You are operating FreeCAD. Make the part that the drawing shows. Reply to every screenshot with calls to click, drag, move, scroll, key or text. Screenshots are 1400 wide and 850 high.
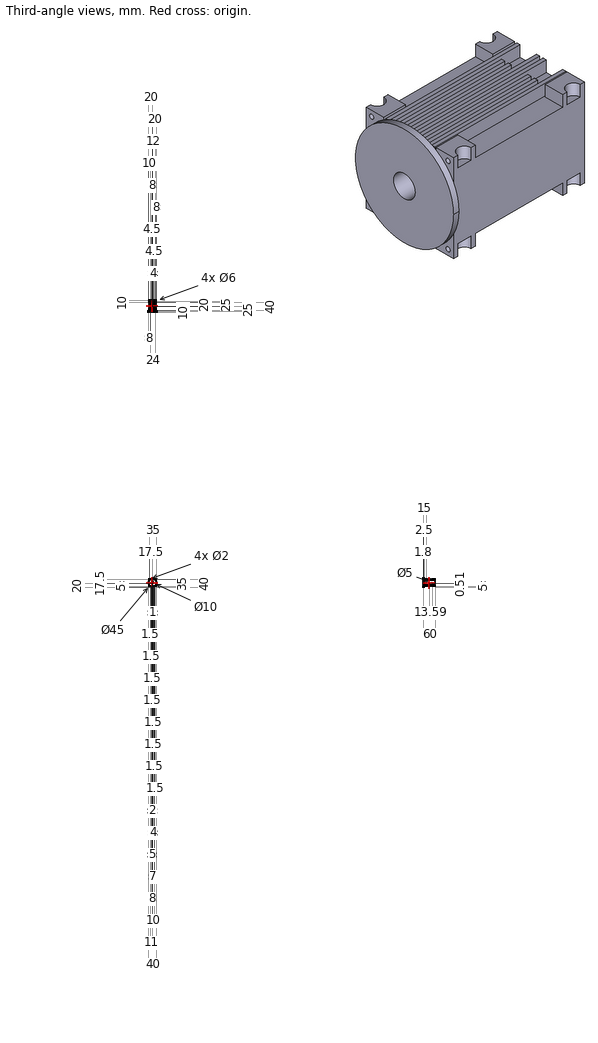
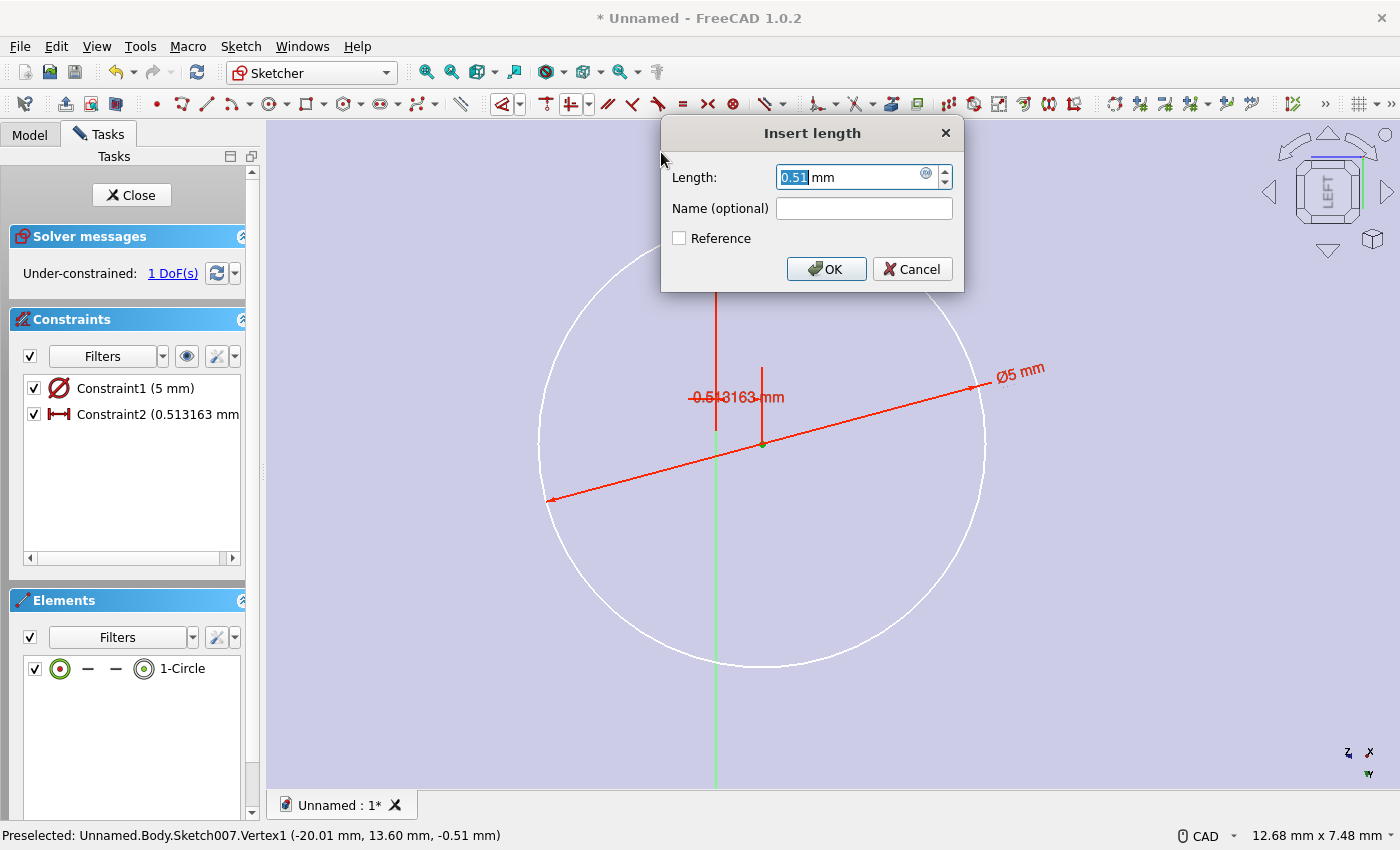
text(0.51)
key(Return)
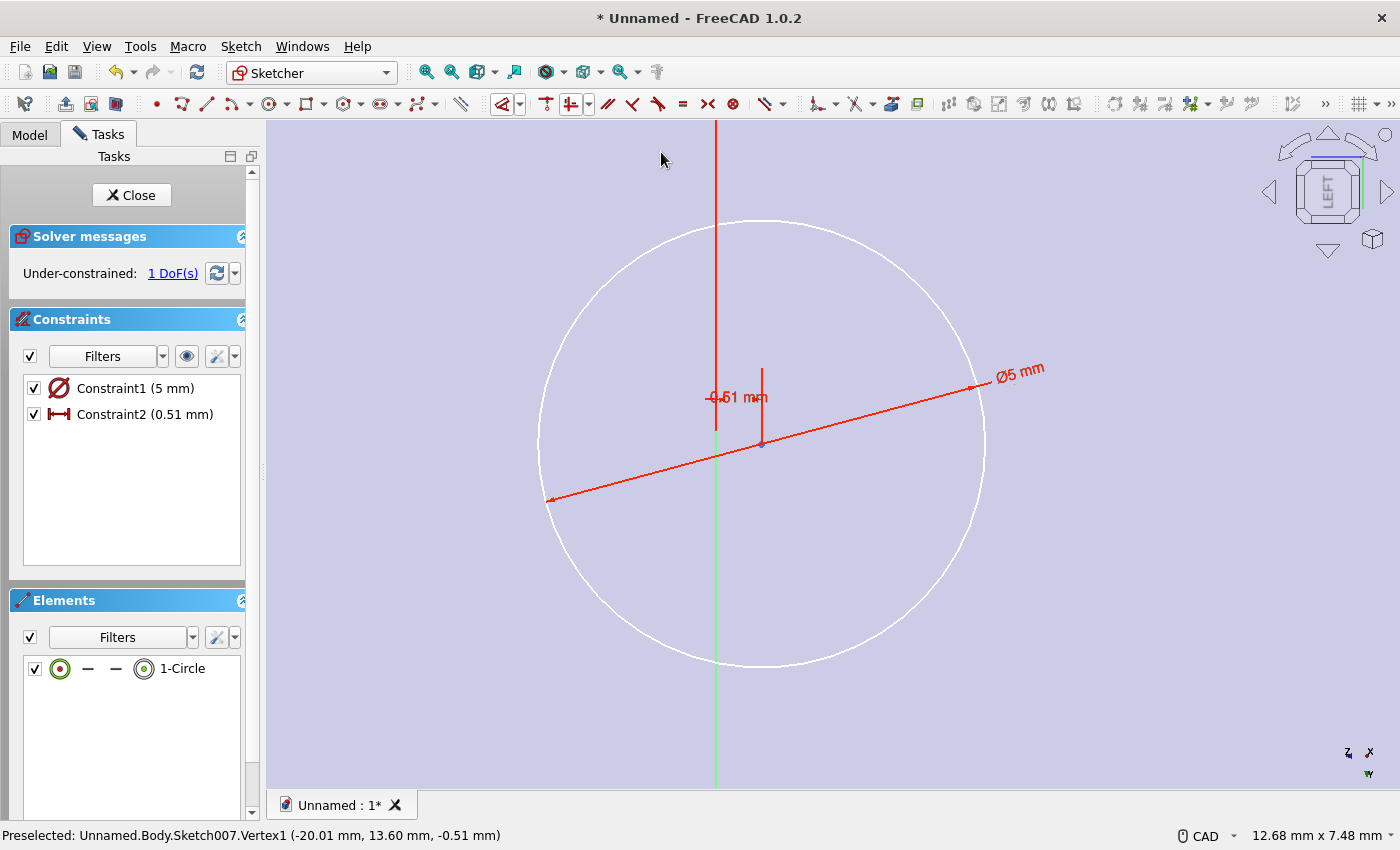
click(762, 444)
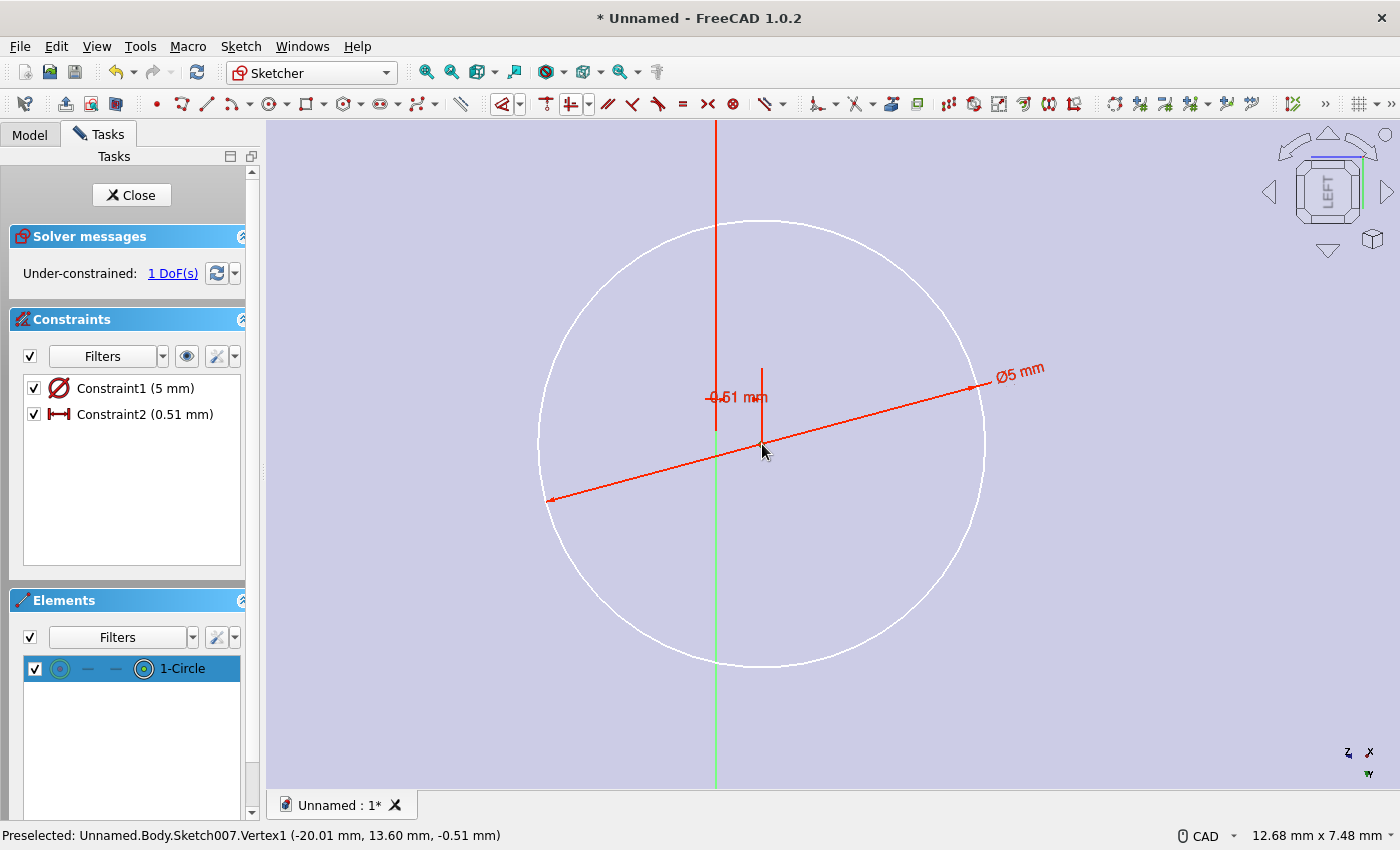
click(520, 104)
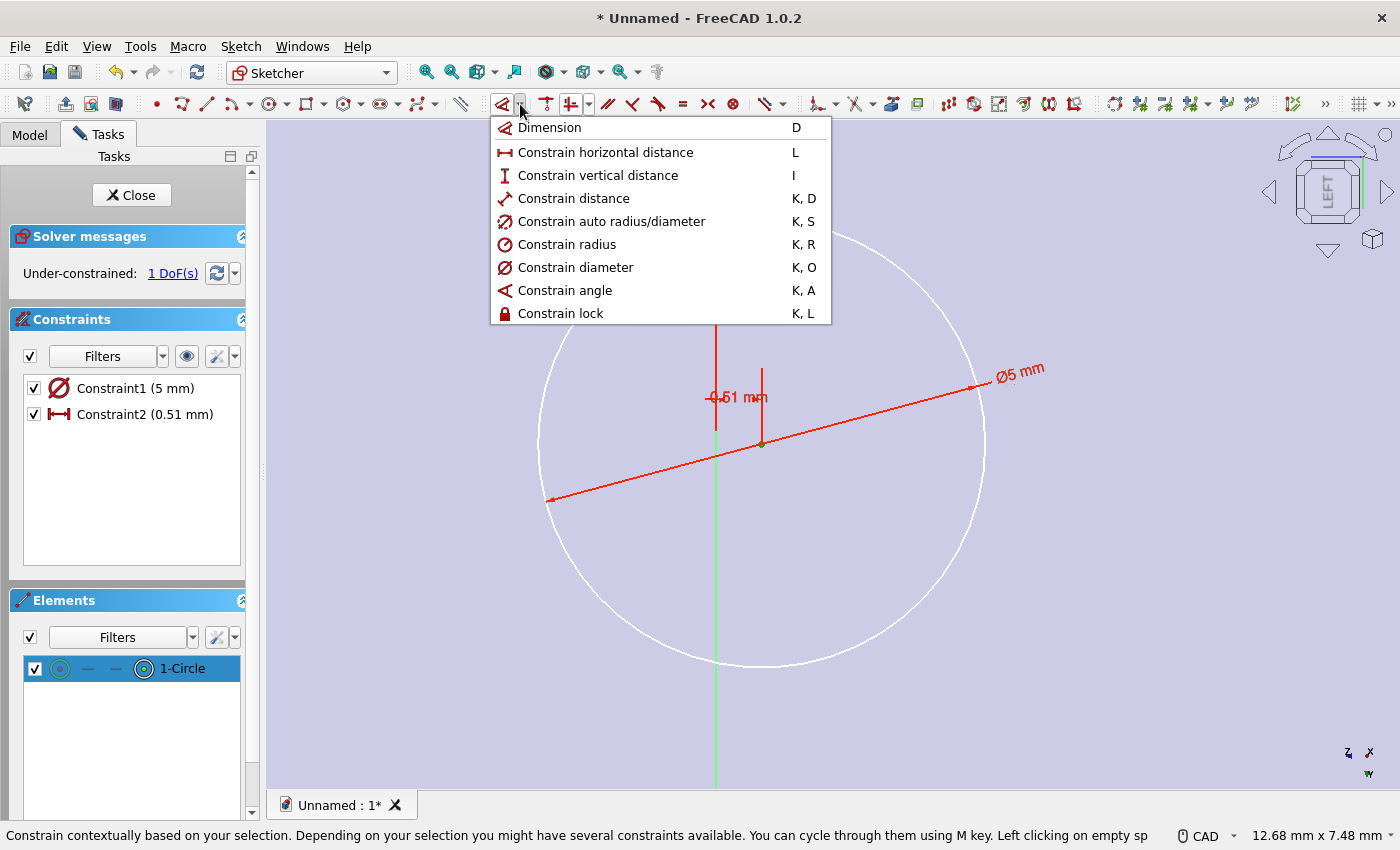
click(661, 176)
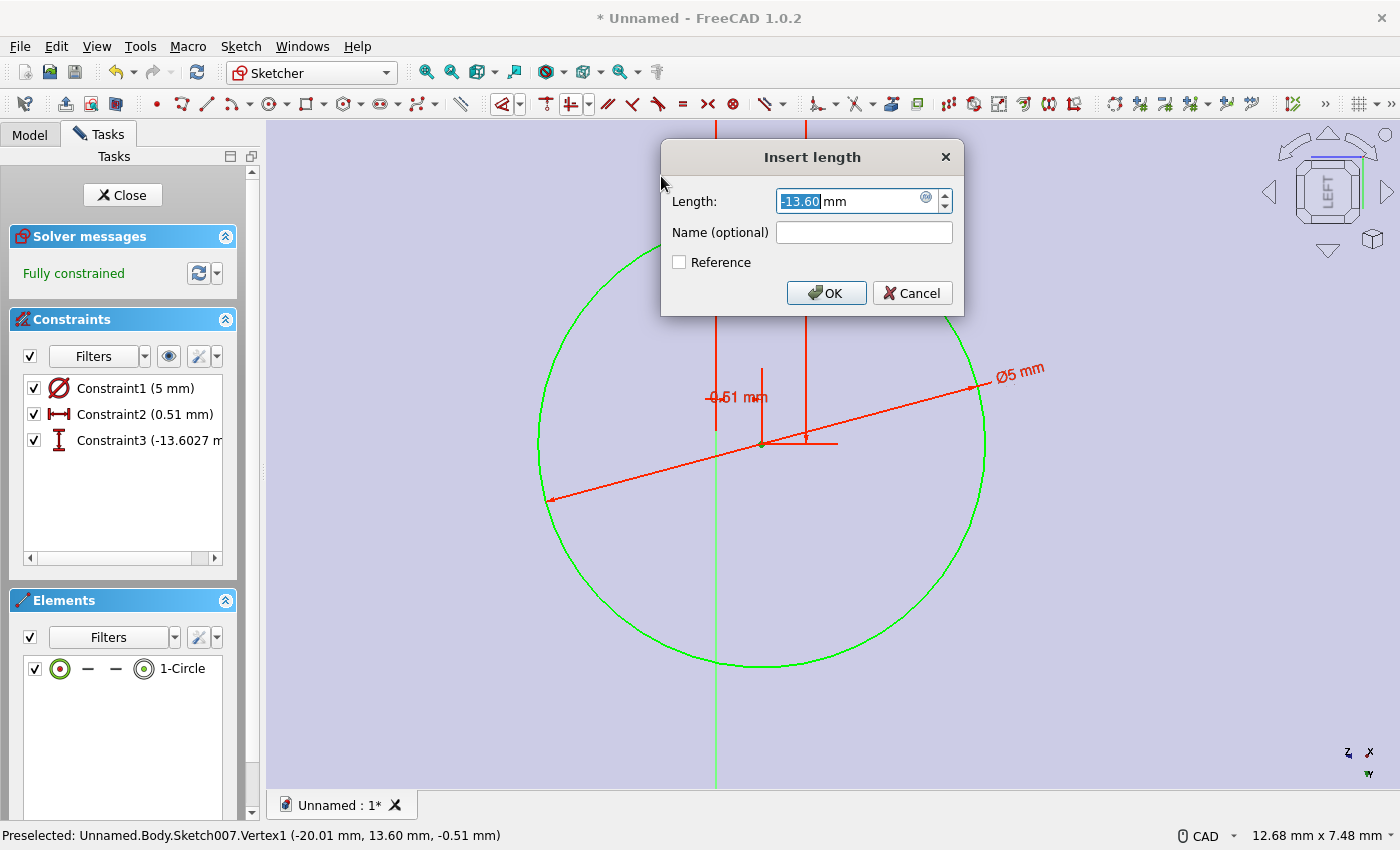
text(-13.59)
key(Return)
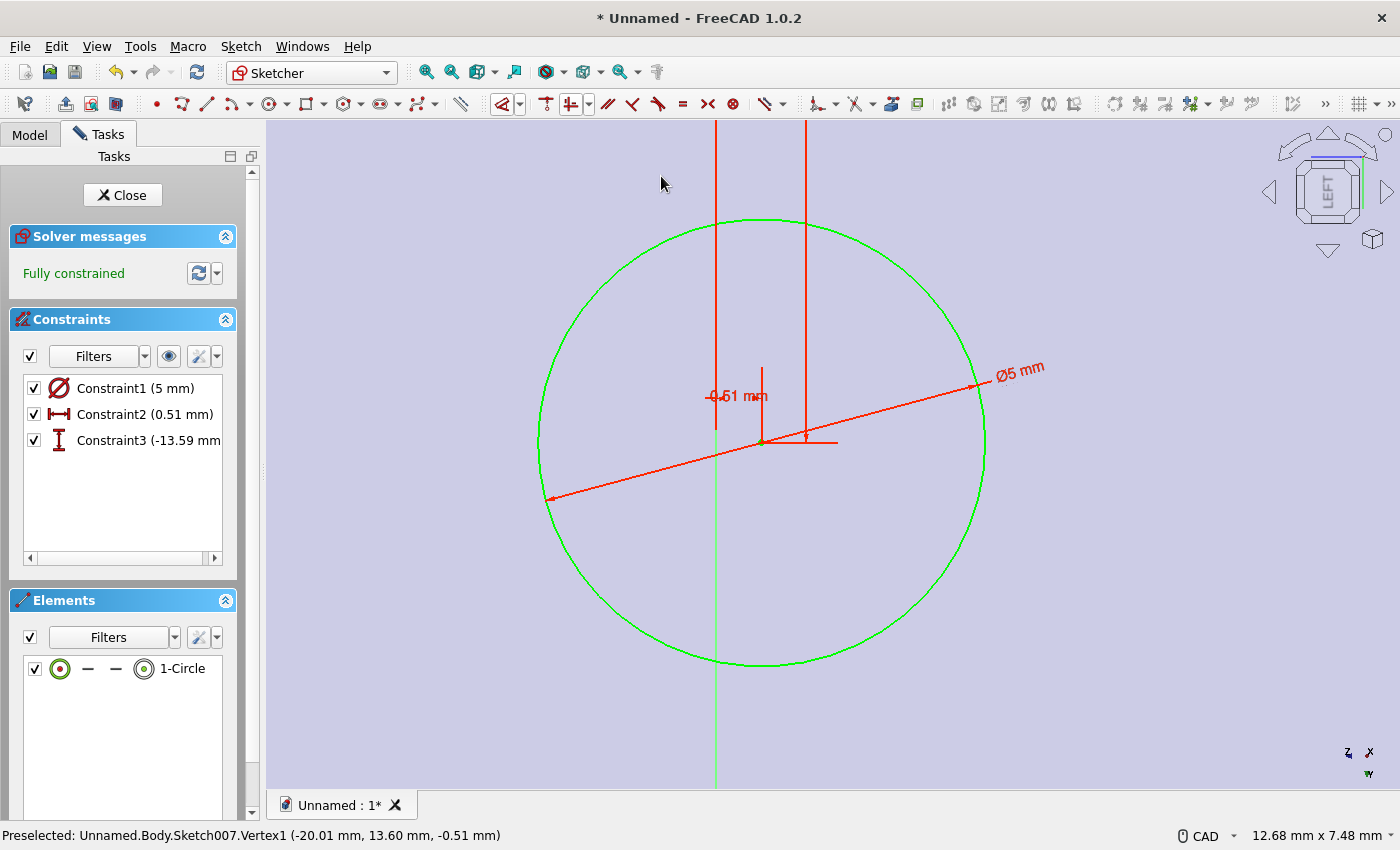
click(123, 195)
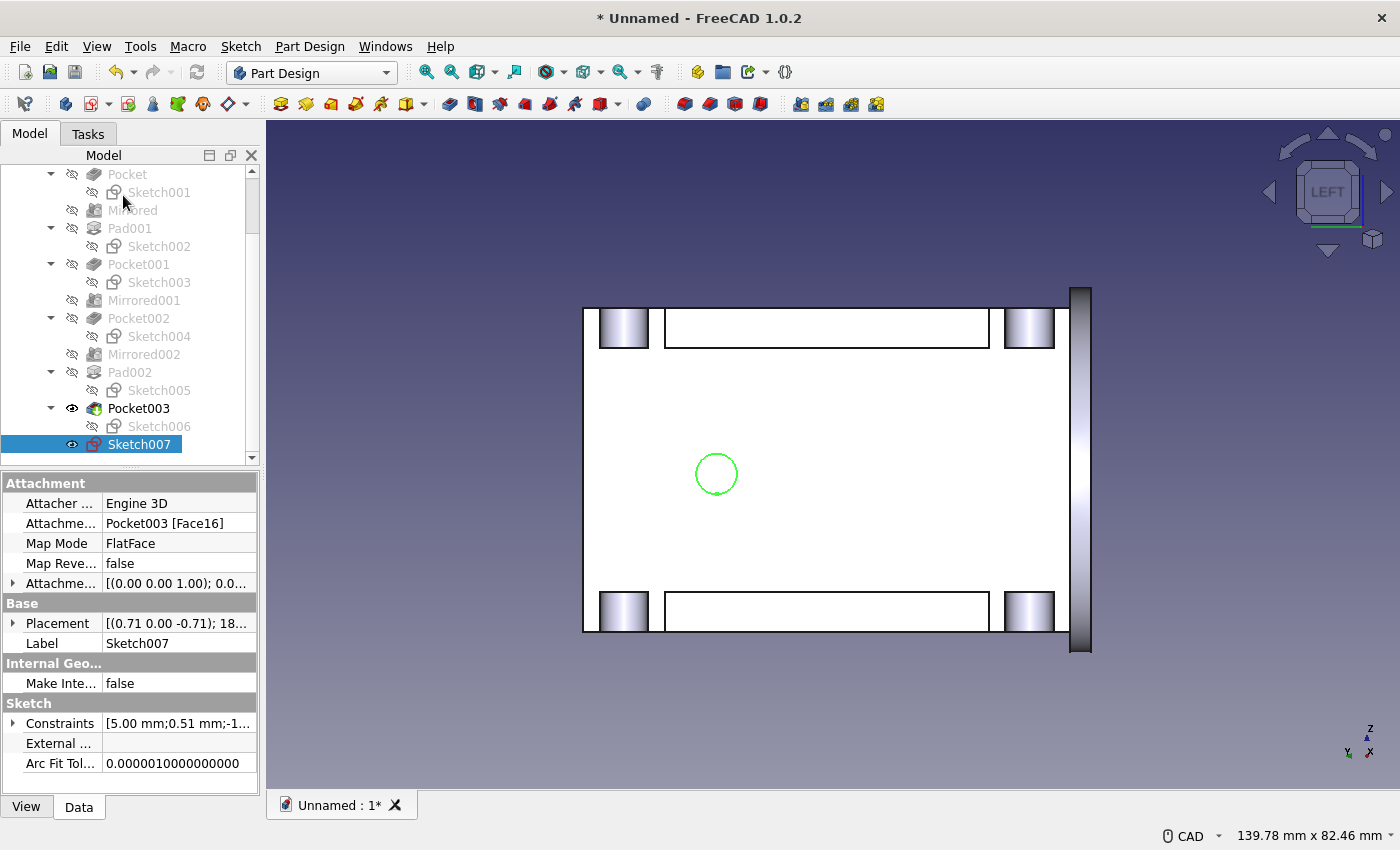
click(450, 104)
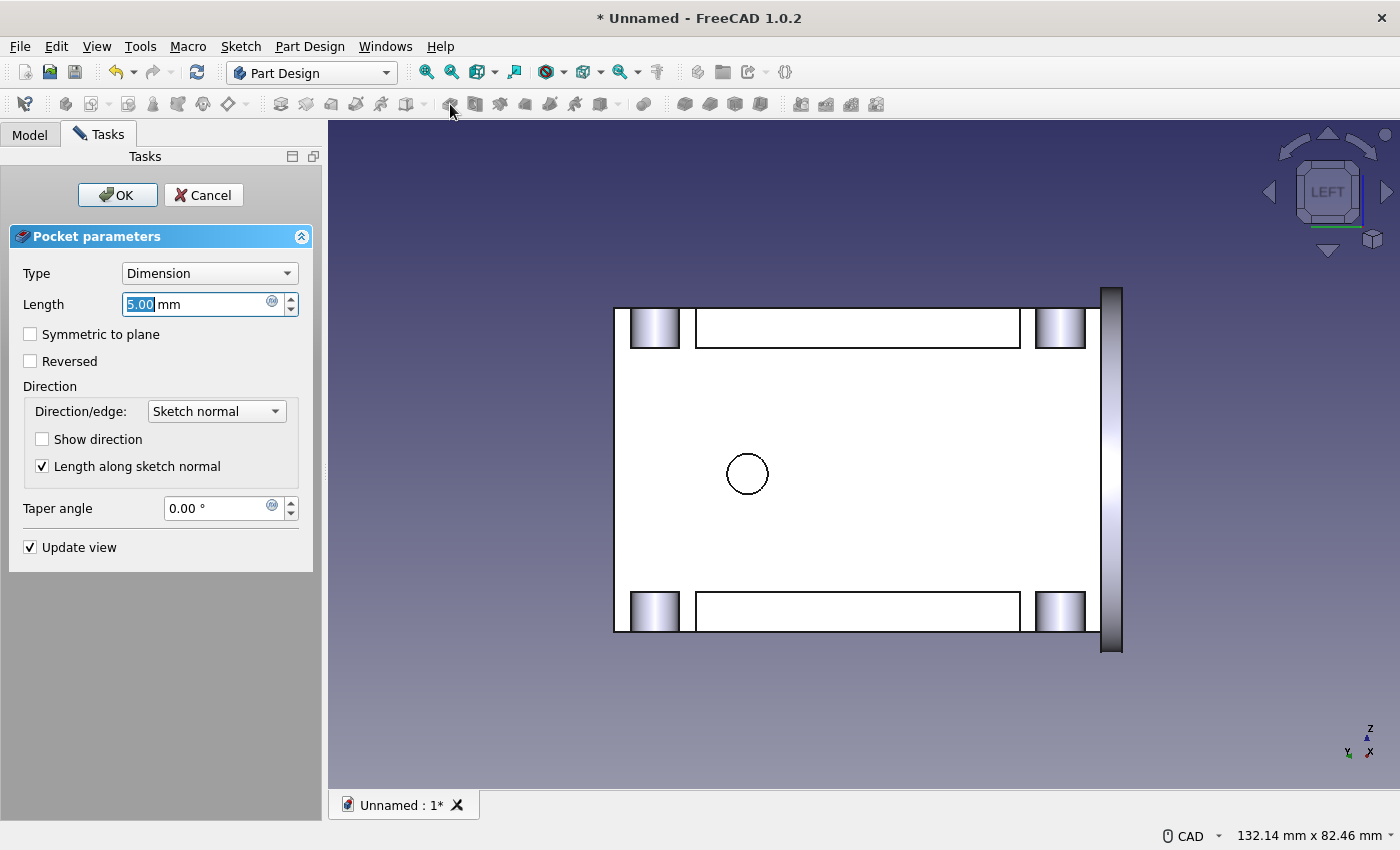
text(10)
key(Tab)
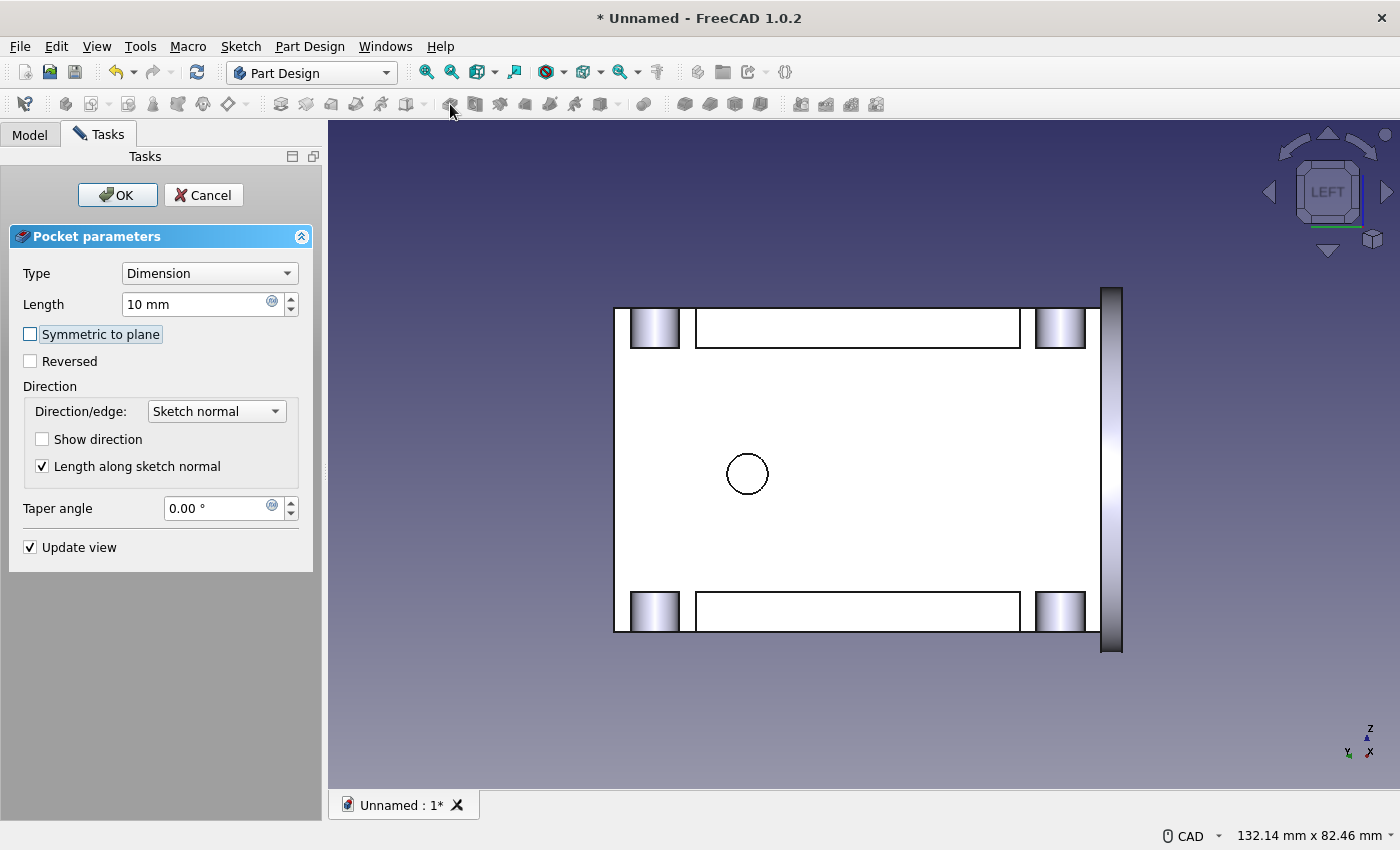
click(118, 195)